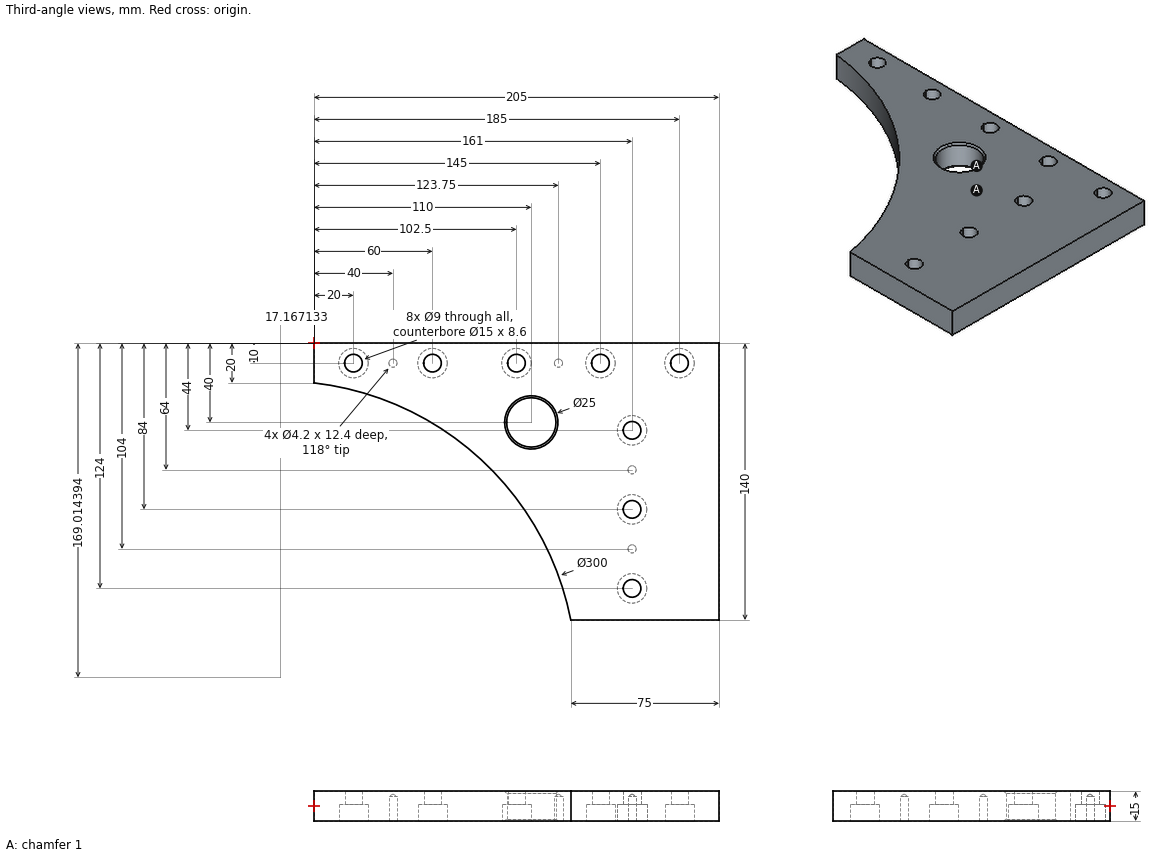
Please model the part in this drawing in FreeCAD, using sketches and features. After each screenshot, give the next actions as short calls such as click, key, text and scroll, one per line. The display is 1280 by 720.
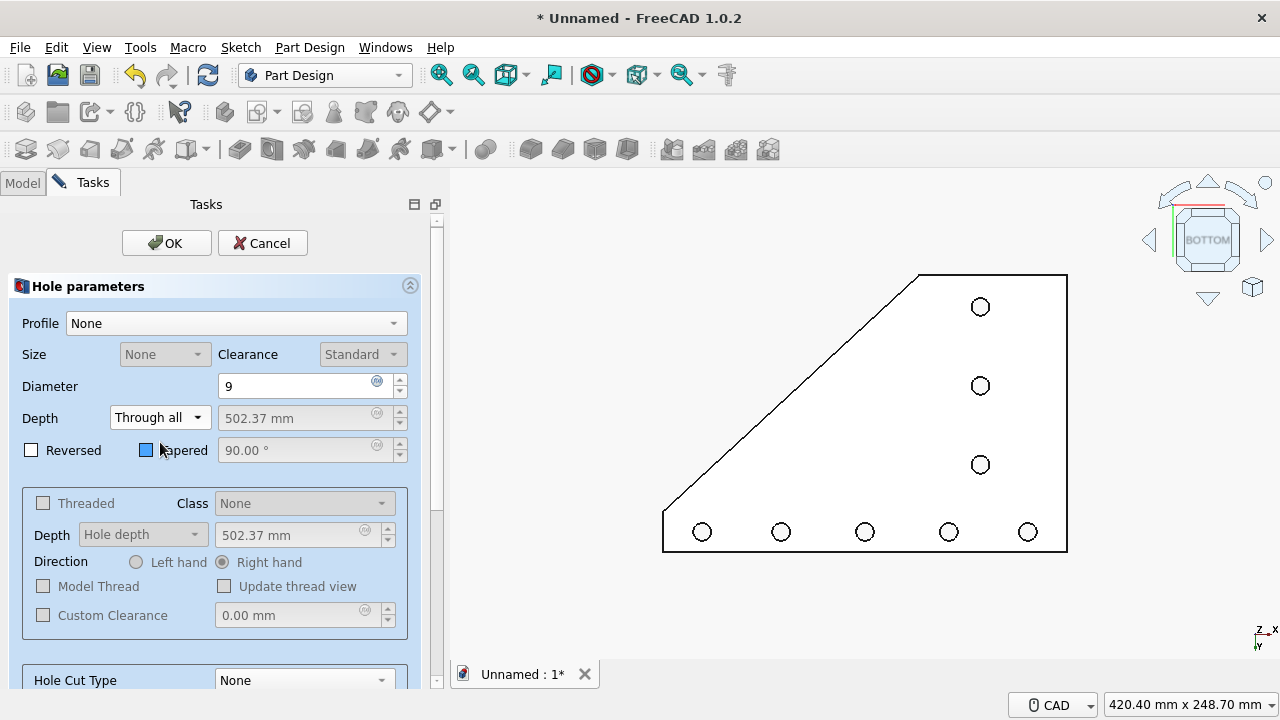
scroll(437, 451, down, 2)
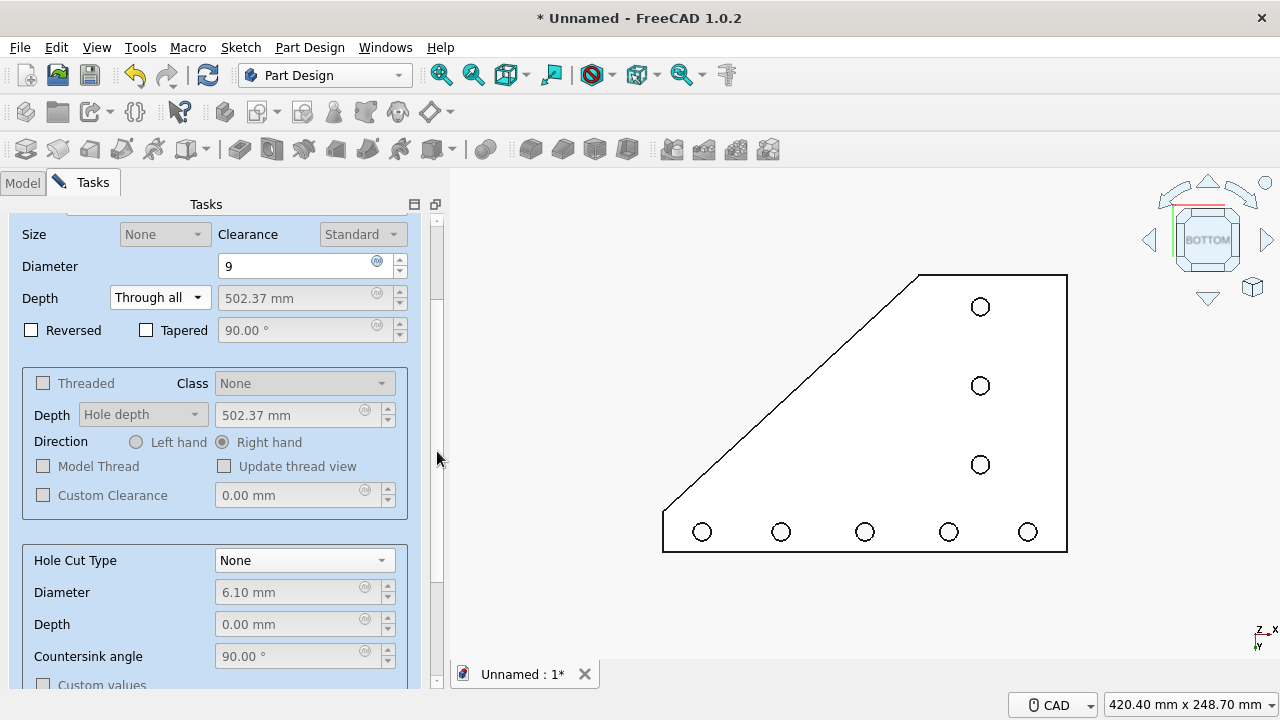
click(306, 560)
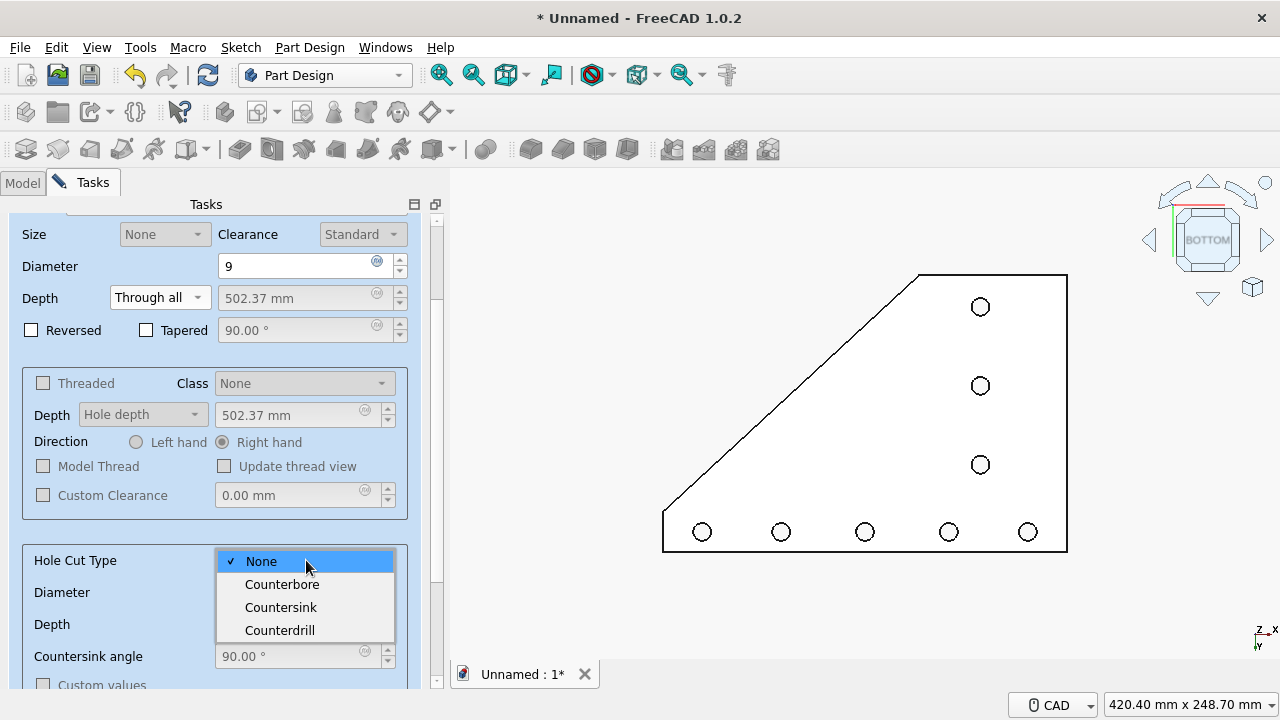
click(304, 584)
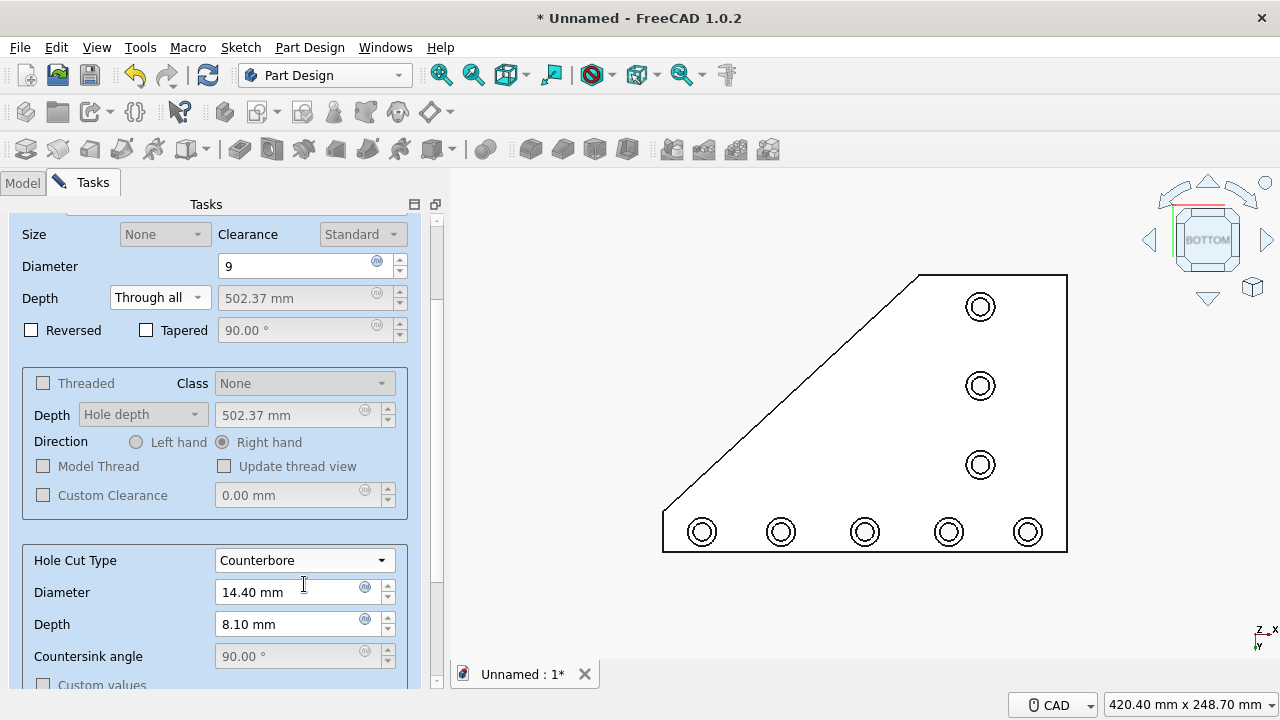
triple_click(298, 592)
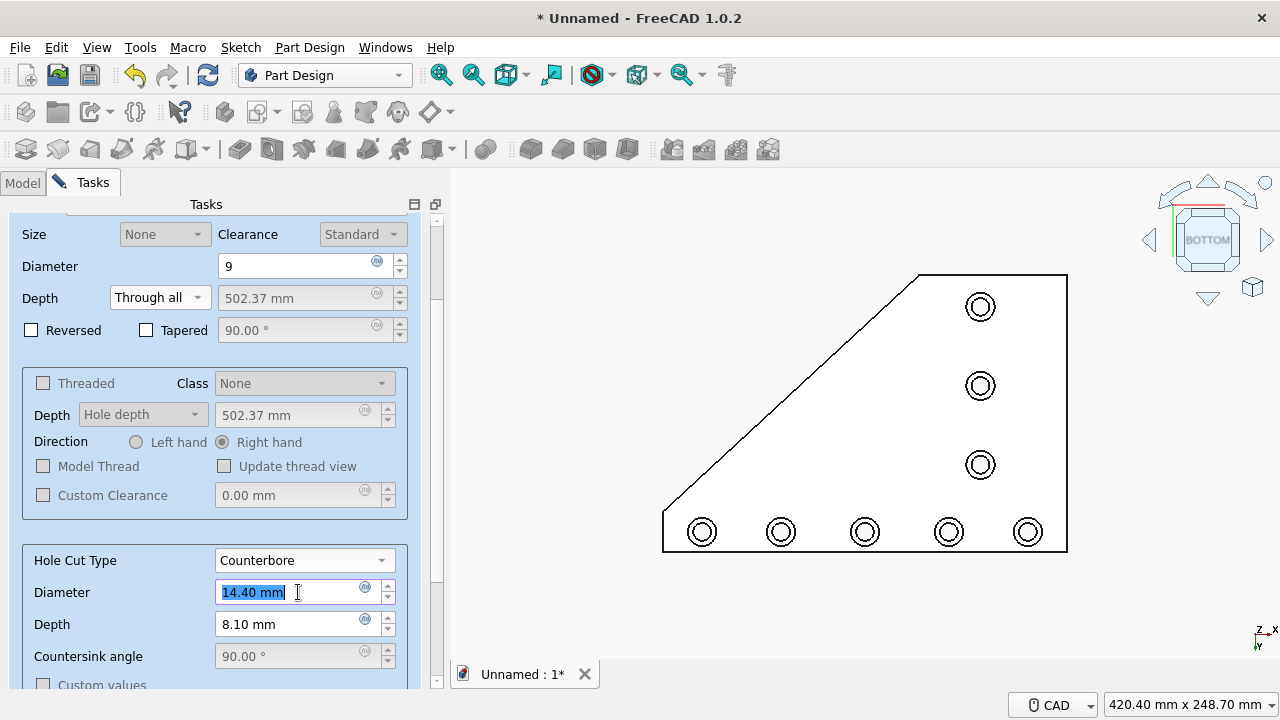
text(15)
key(Tab)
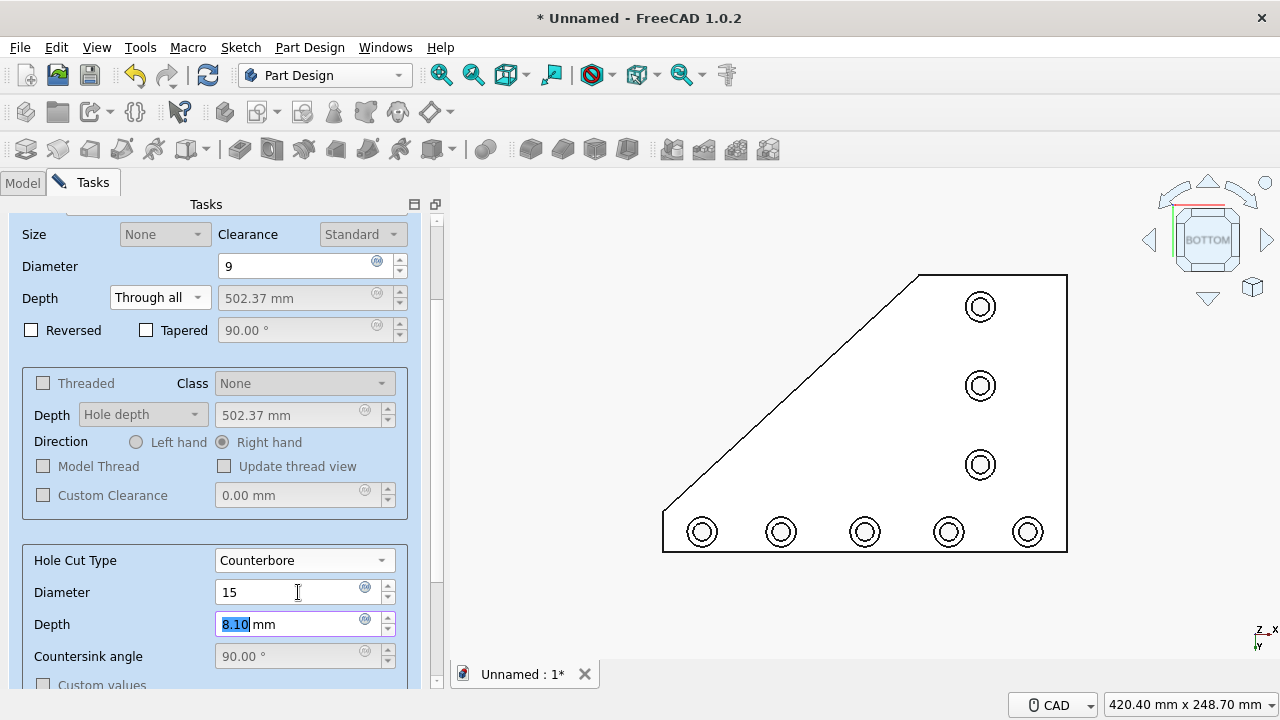
text(8.6)
key(Tab)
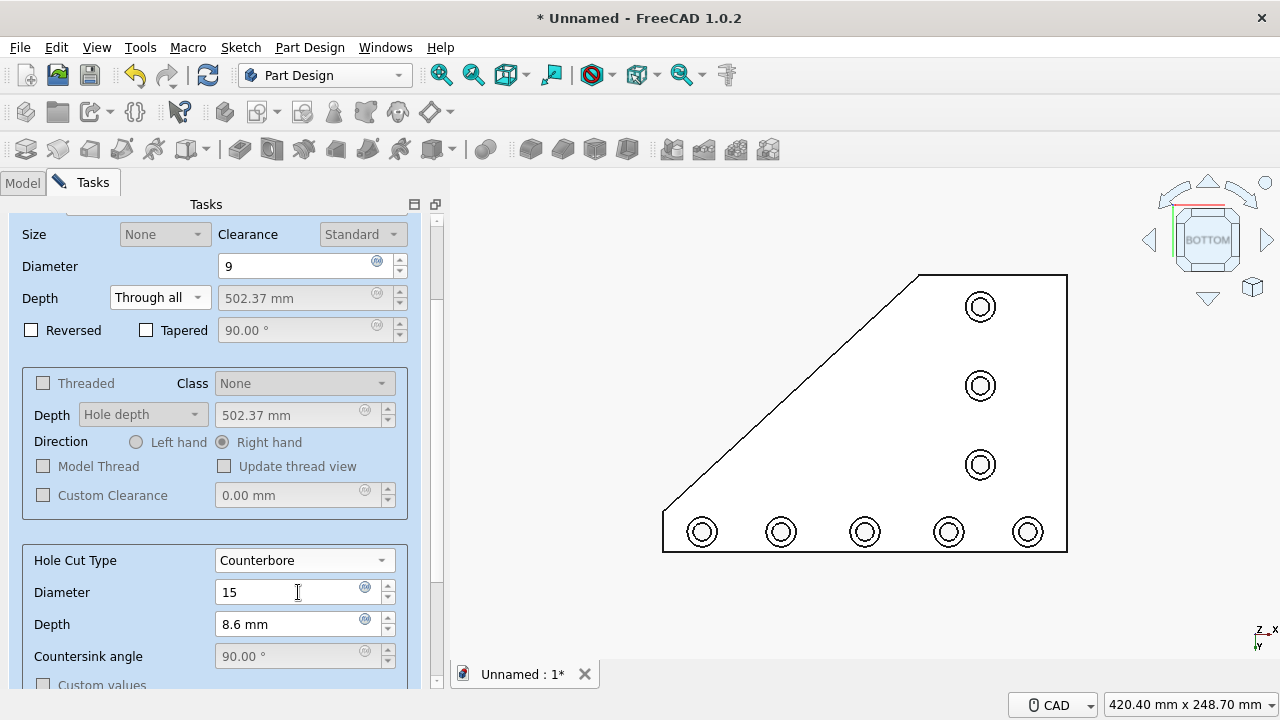
scroll(437, 451, up, 3)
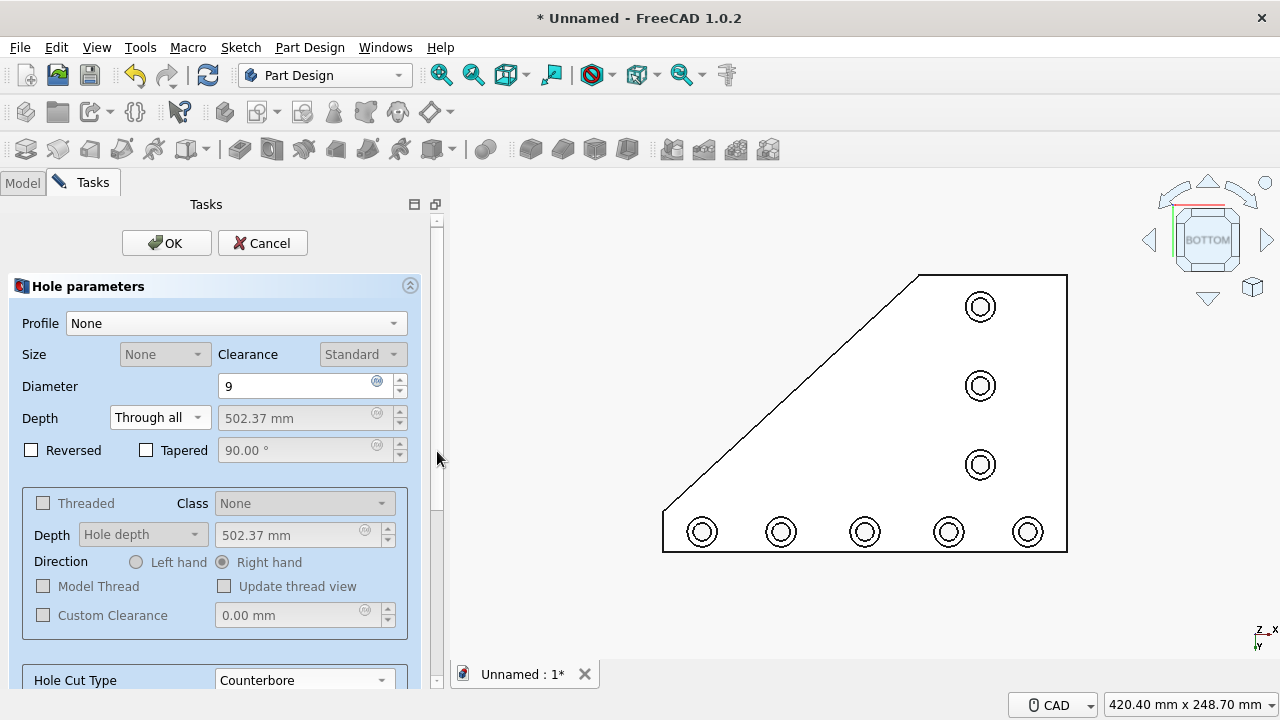
click(167, 243)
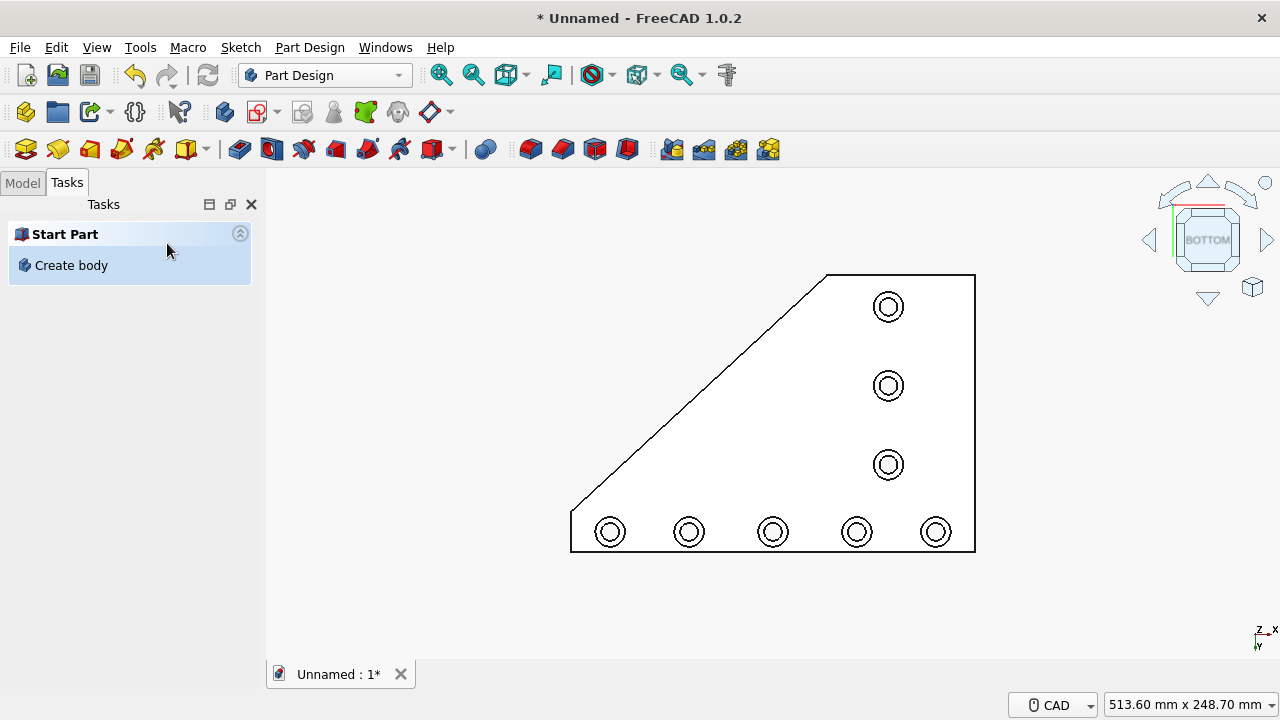
click(773, 412)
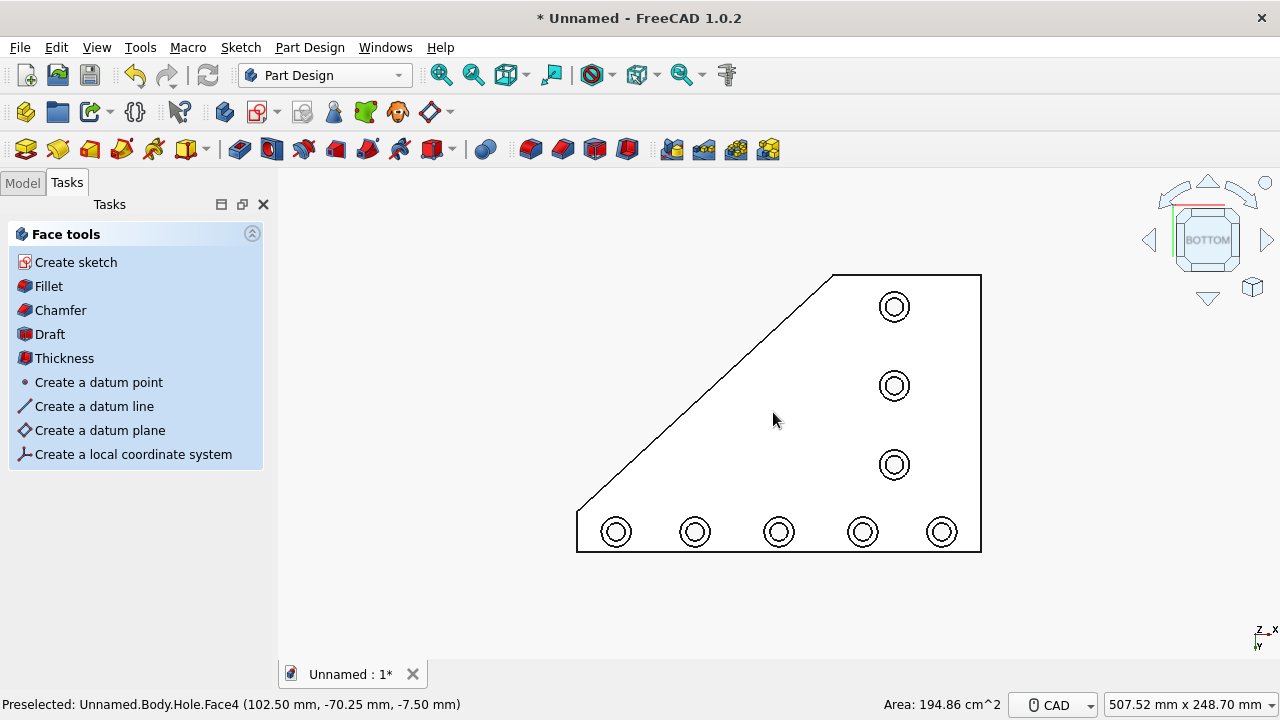
click(258, 112)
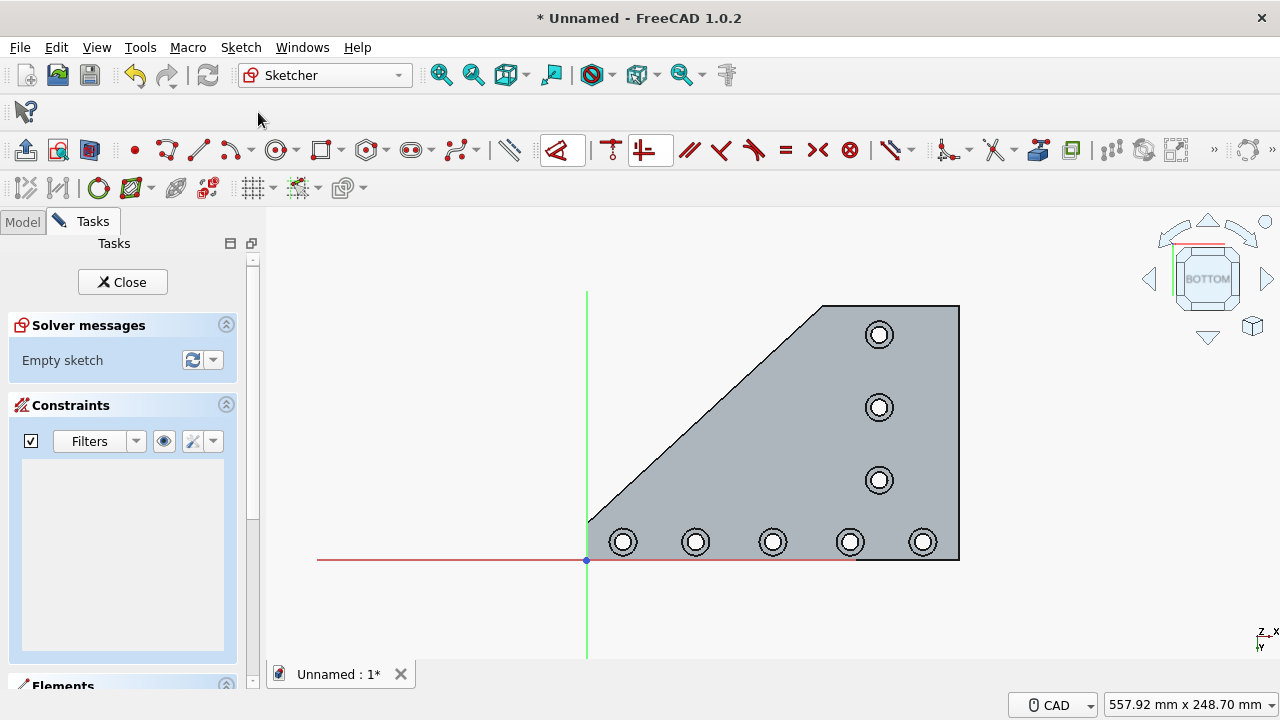
scroll(797, 526, up, 2)